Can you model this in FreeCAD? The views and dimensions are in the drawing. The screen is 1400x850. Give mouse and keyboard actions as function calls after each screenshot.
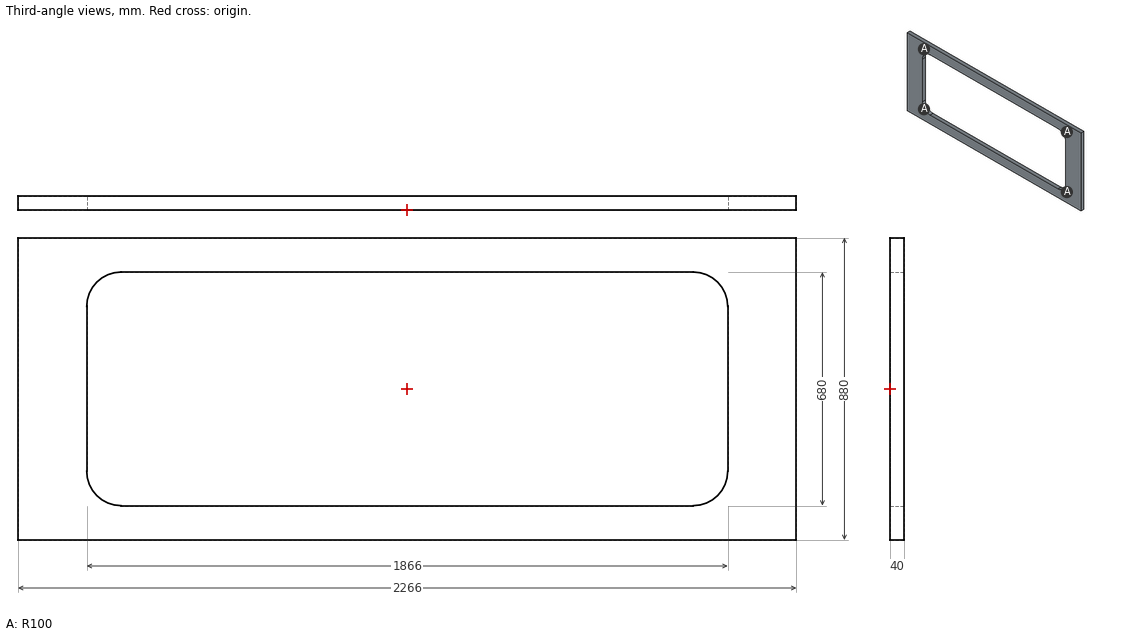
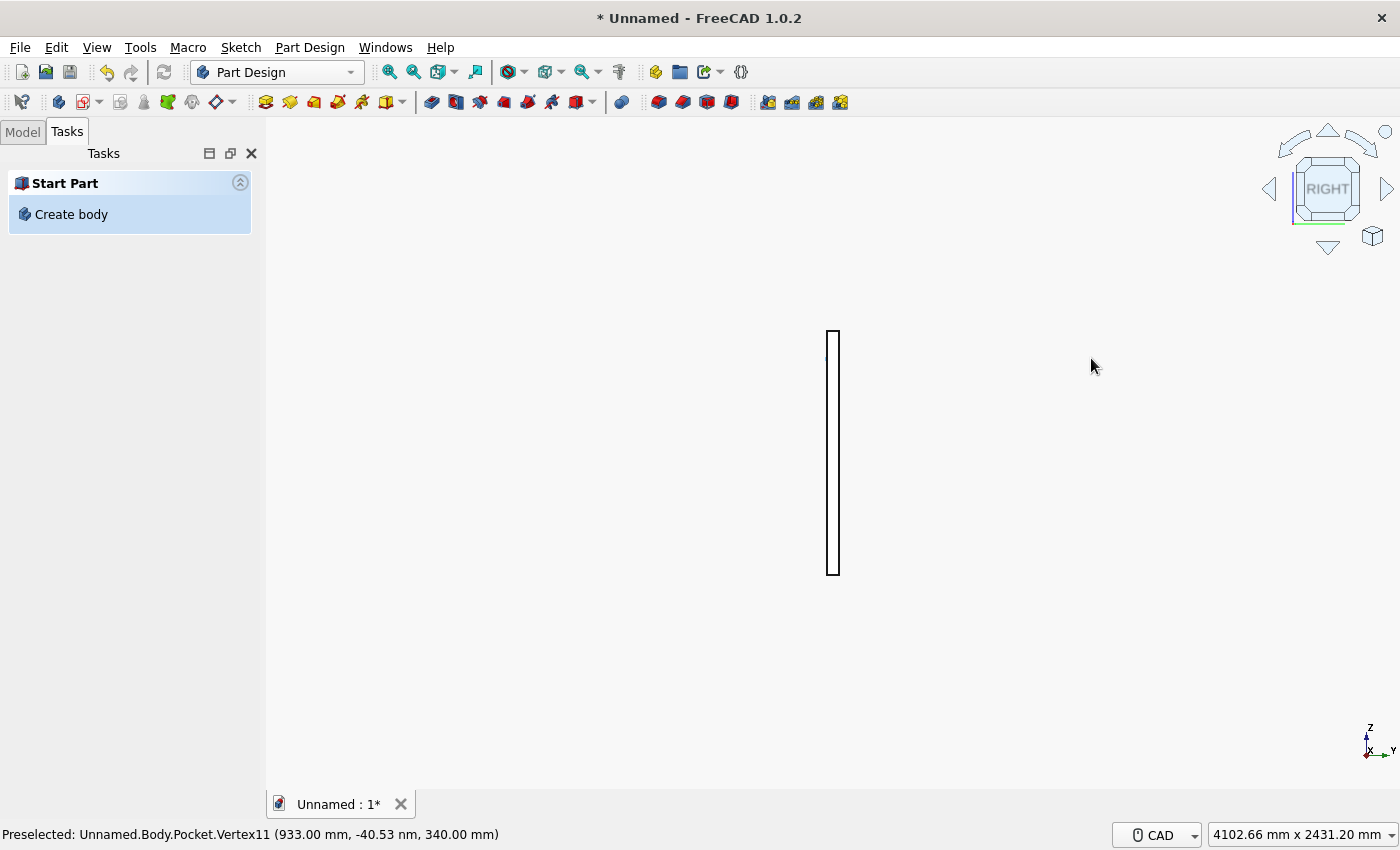
scroll(833, 358, up, 7)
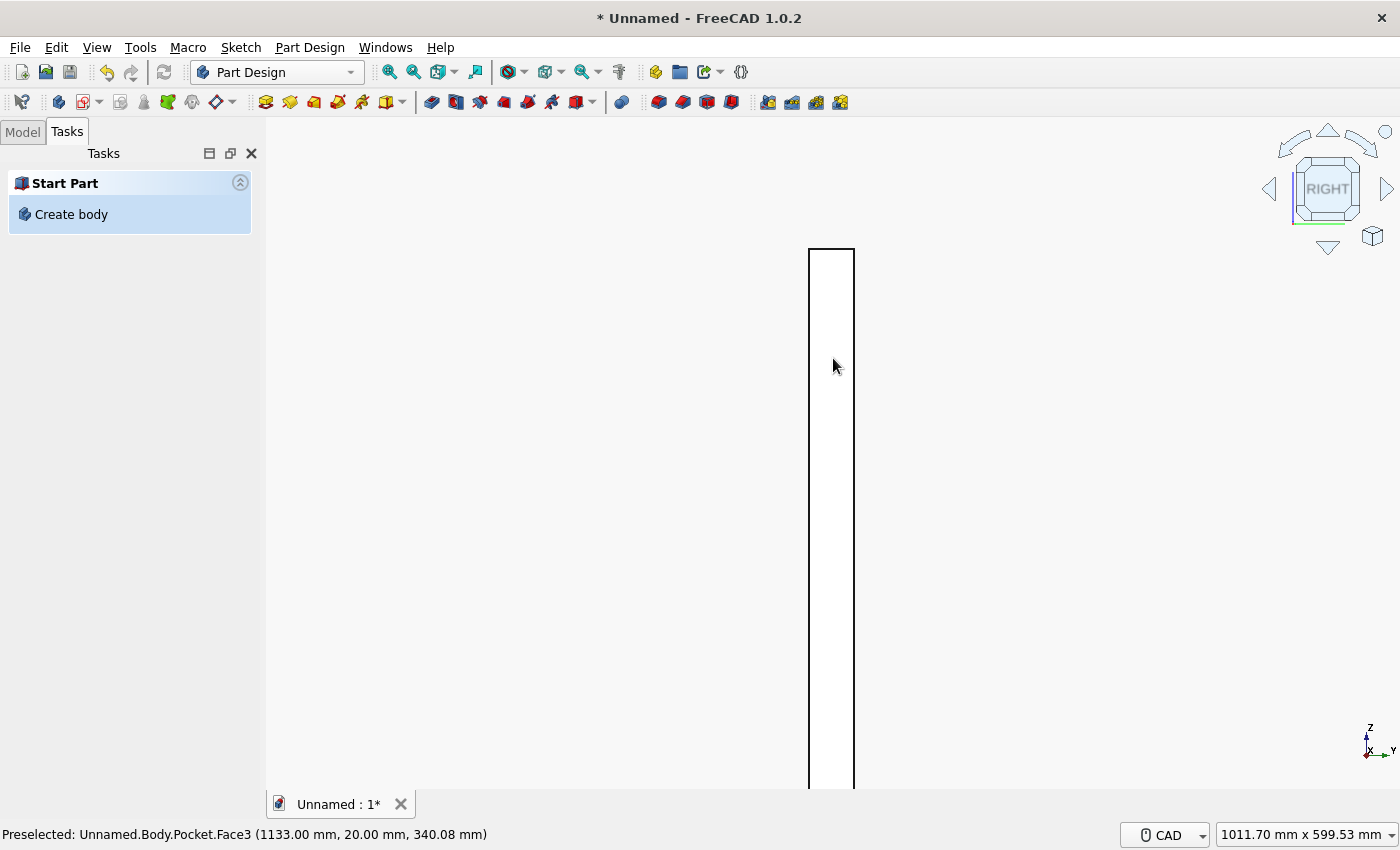
key(v)
key(f)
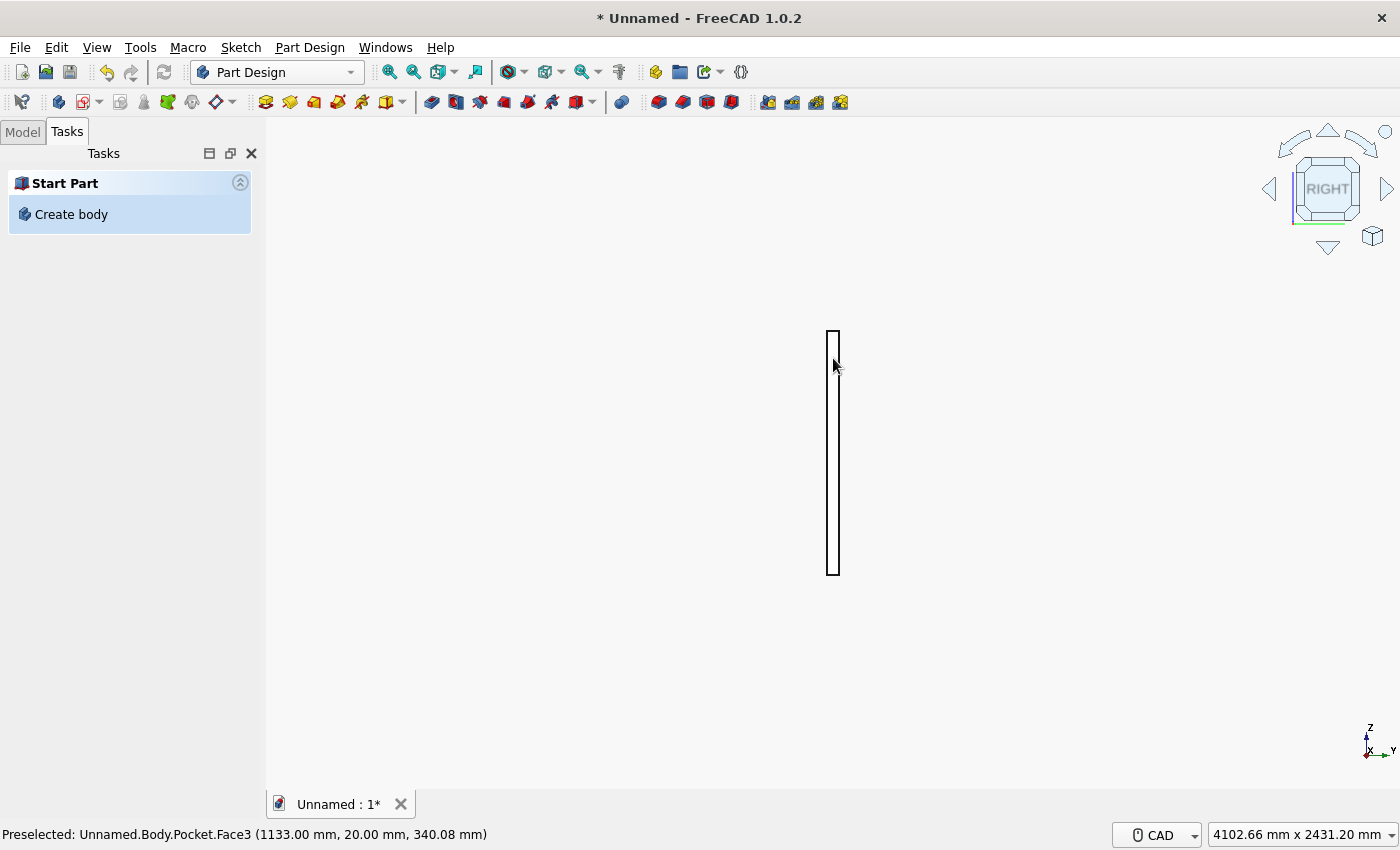
key(5)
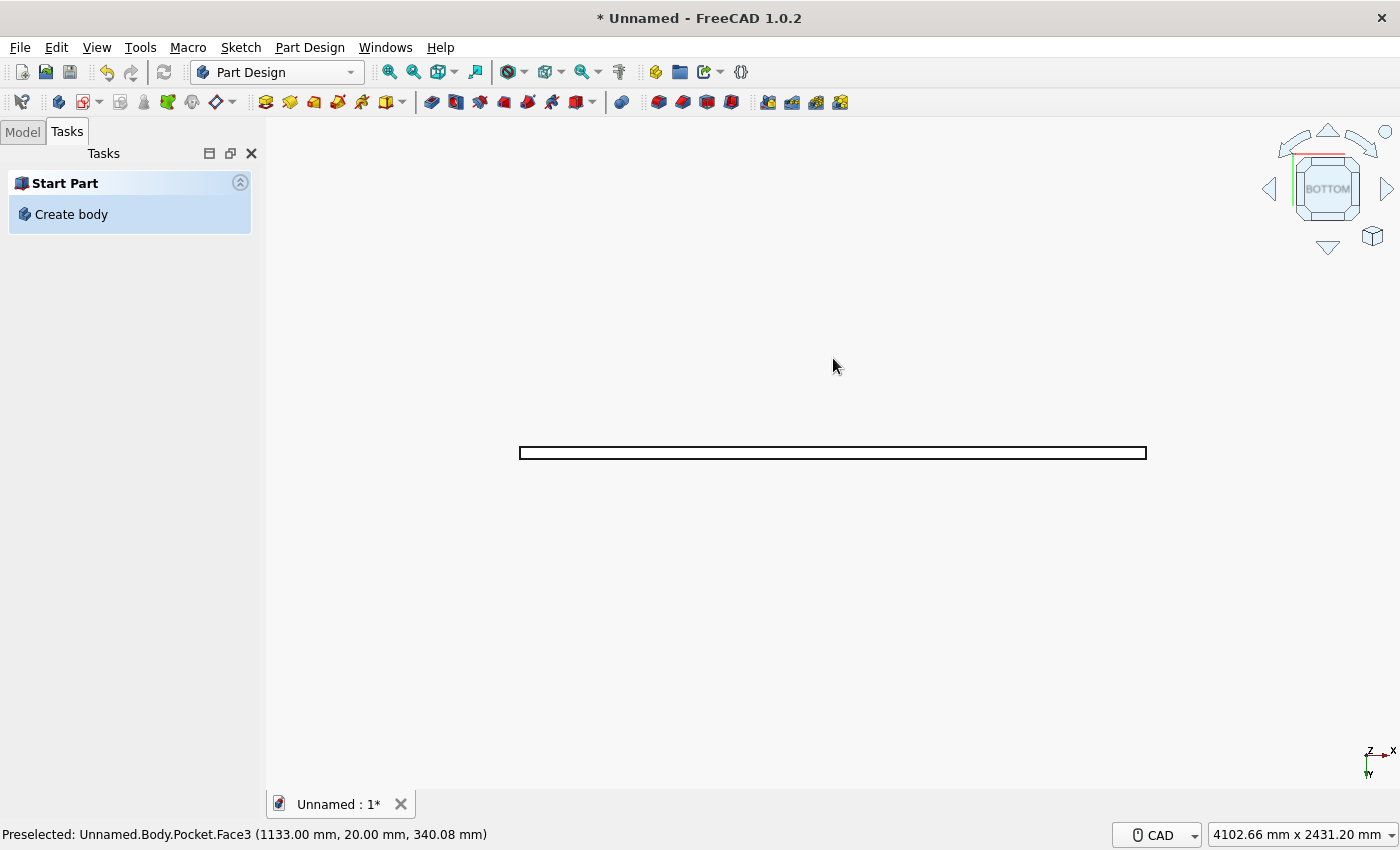
scroll(1091, 452, up, 7)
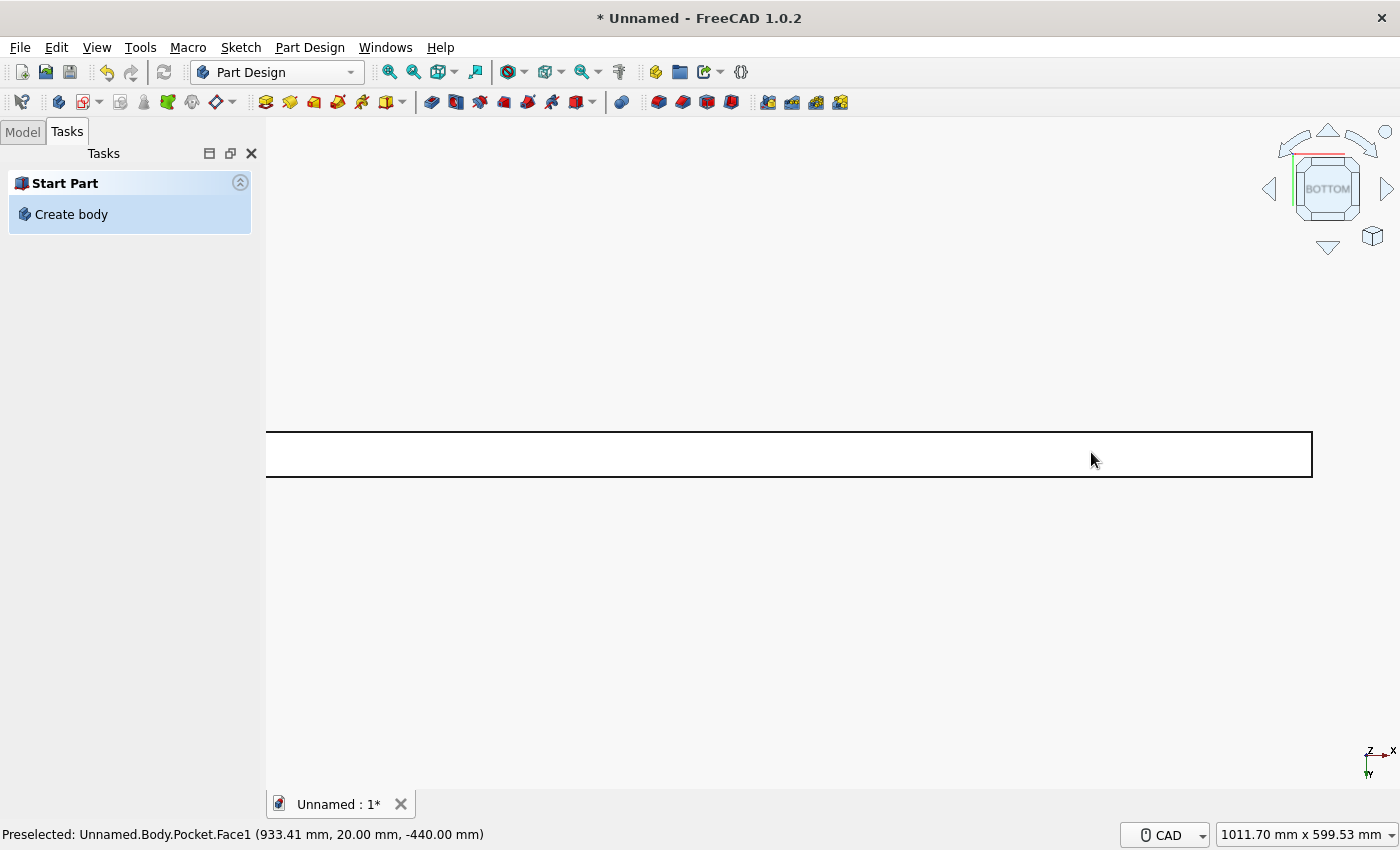
click(390, 72)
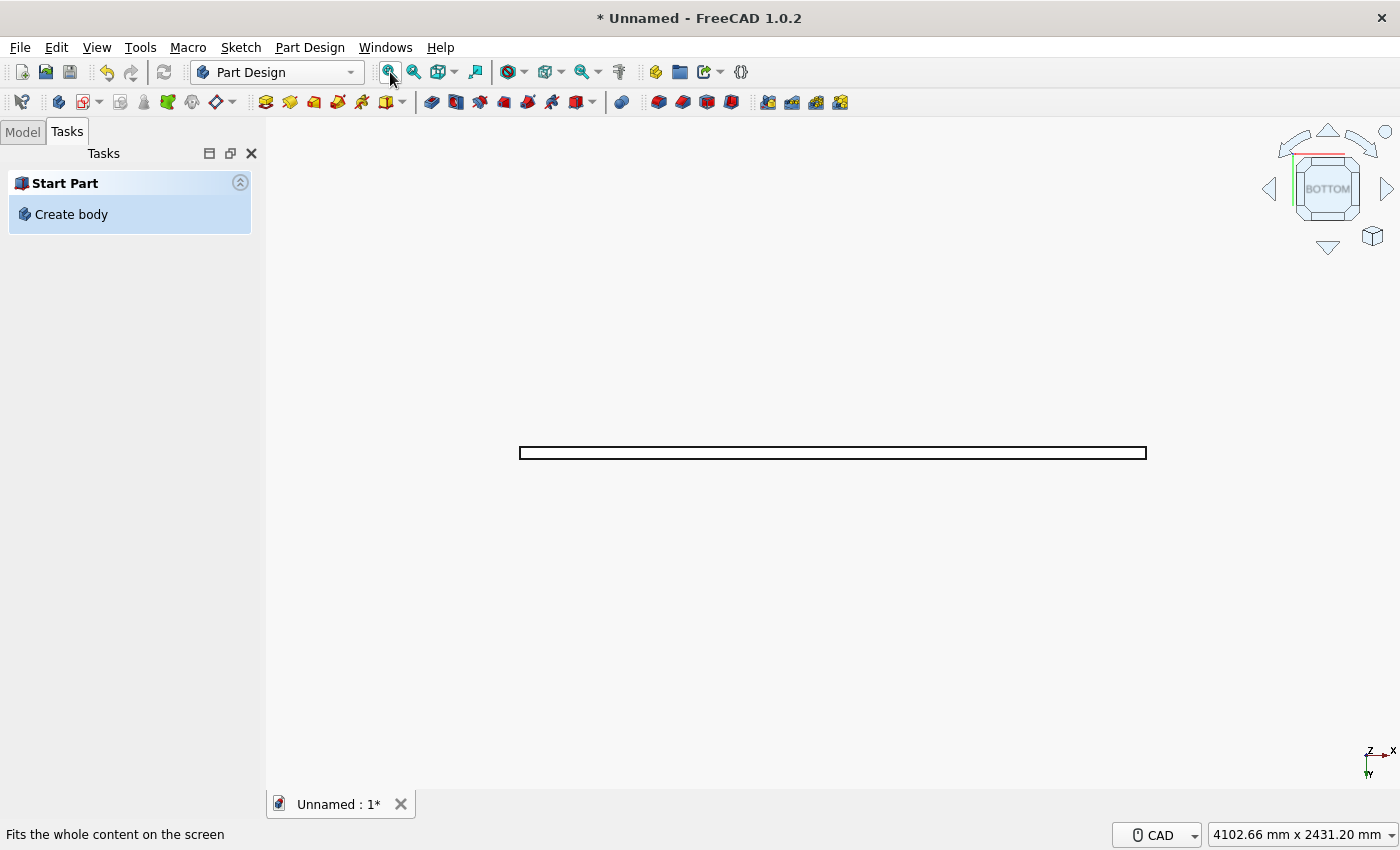
key(4)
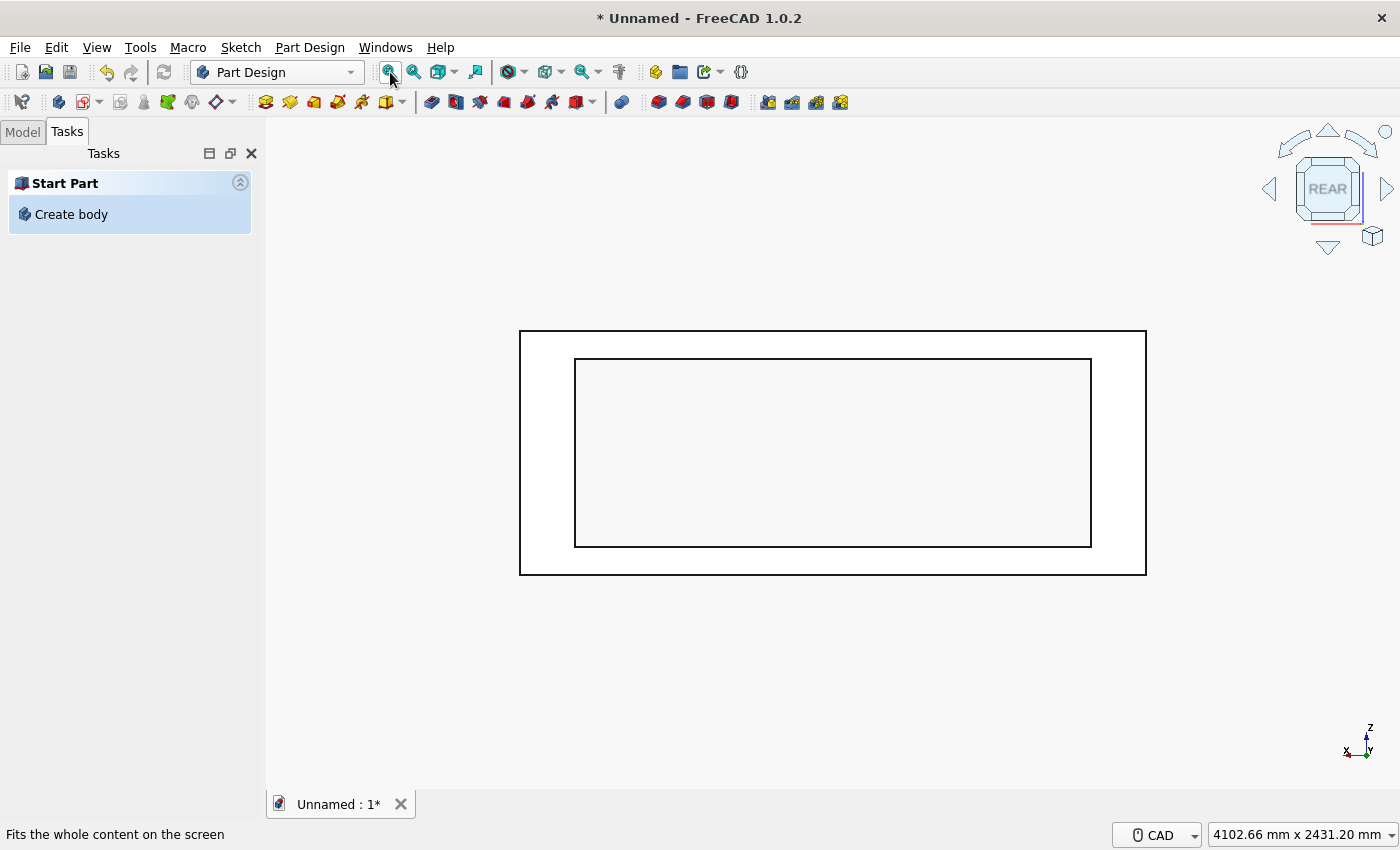
scroll(575, 358, up, 7)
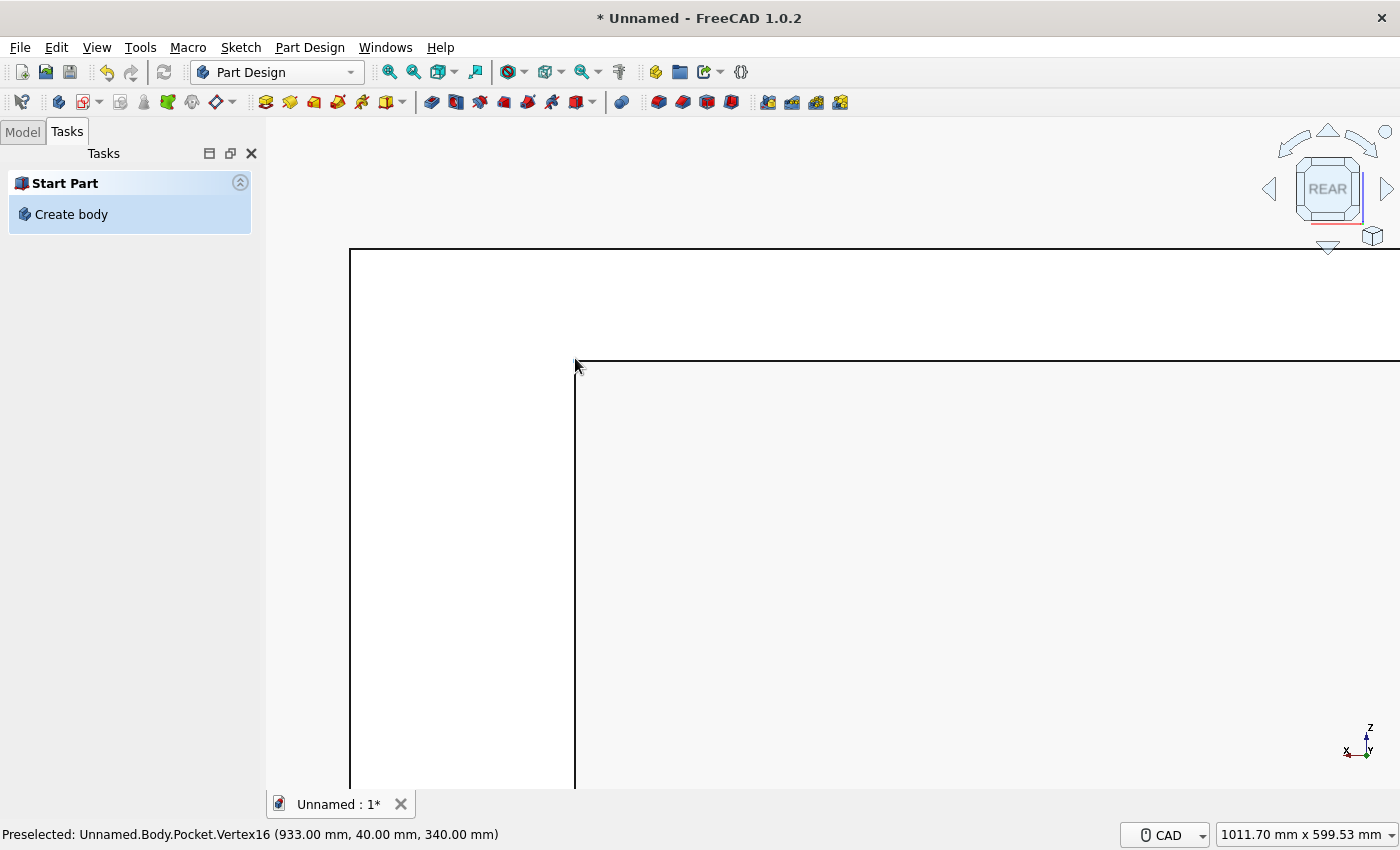
click(390, 72)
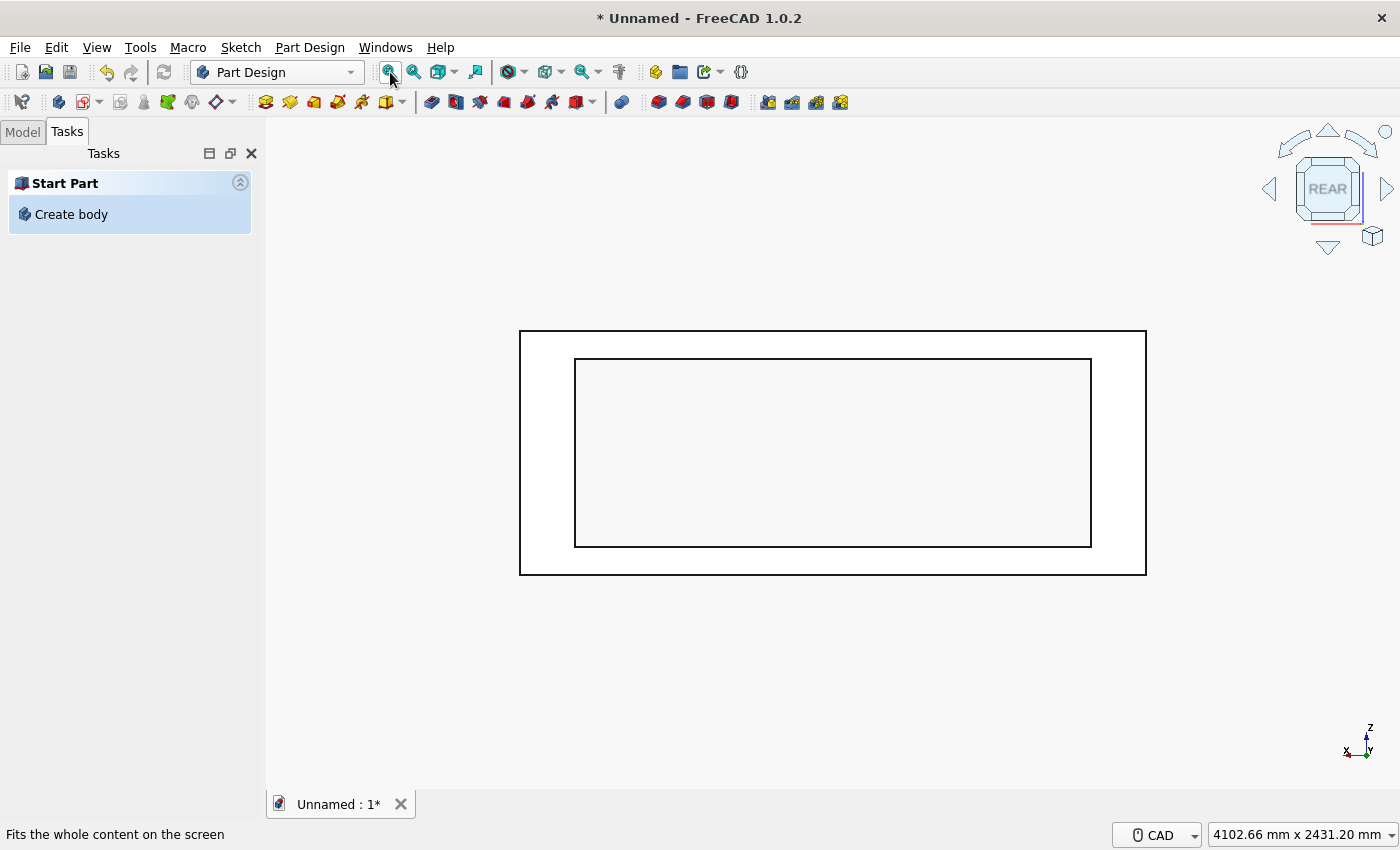
key(6)